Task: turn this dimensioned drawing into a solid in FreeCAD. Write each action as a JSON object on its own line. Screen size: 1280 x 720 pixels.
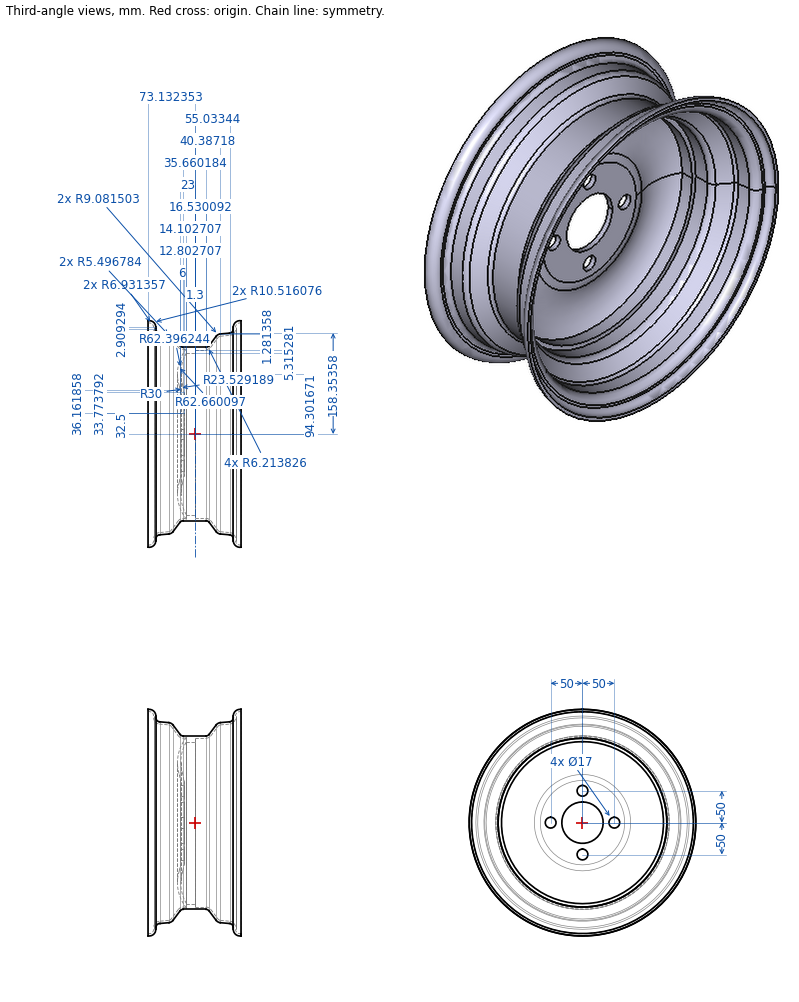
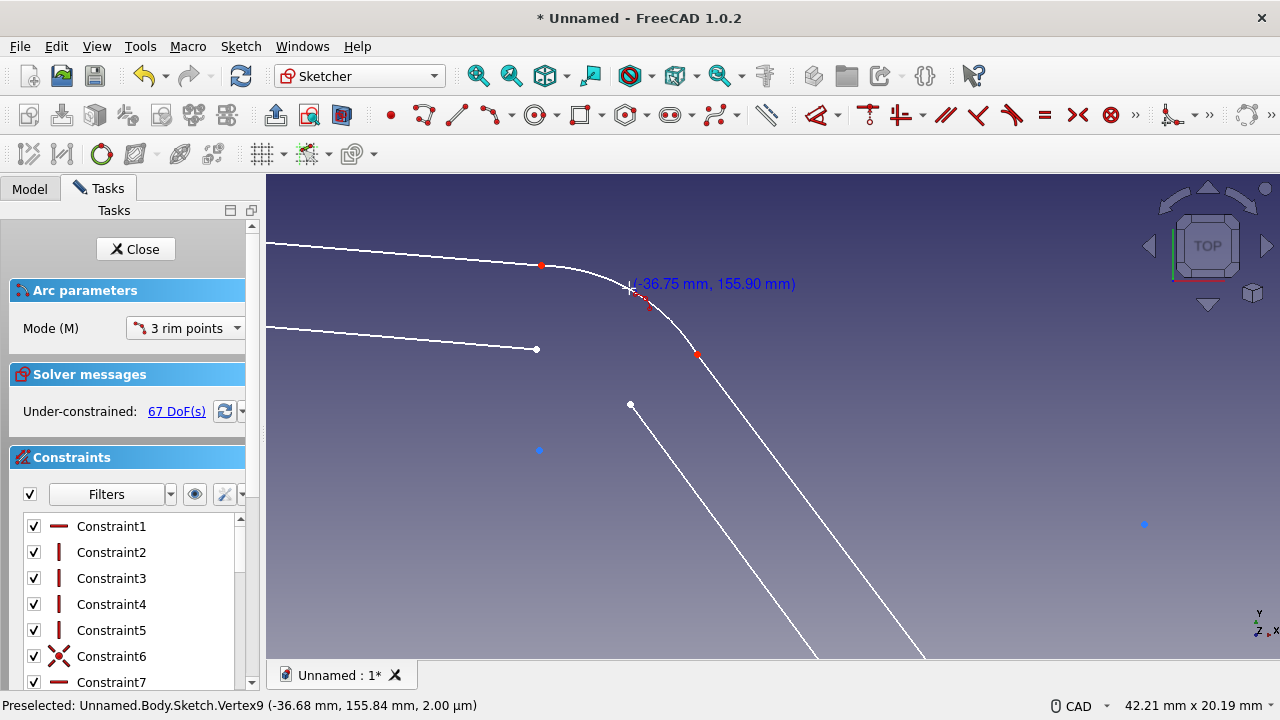
{"action": "scroll", "coordinate": [640, 298], "scroll_direction": "down", "scroll_amount": 13}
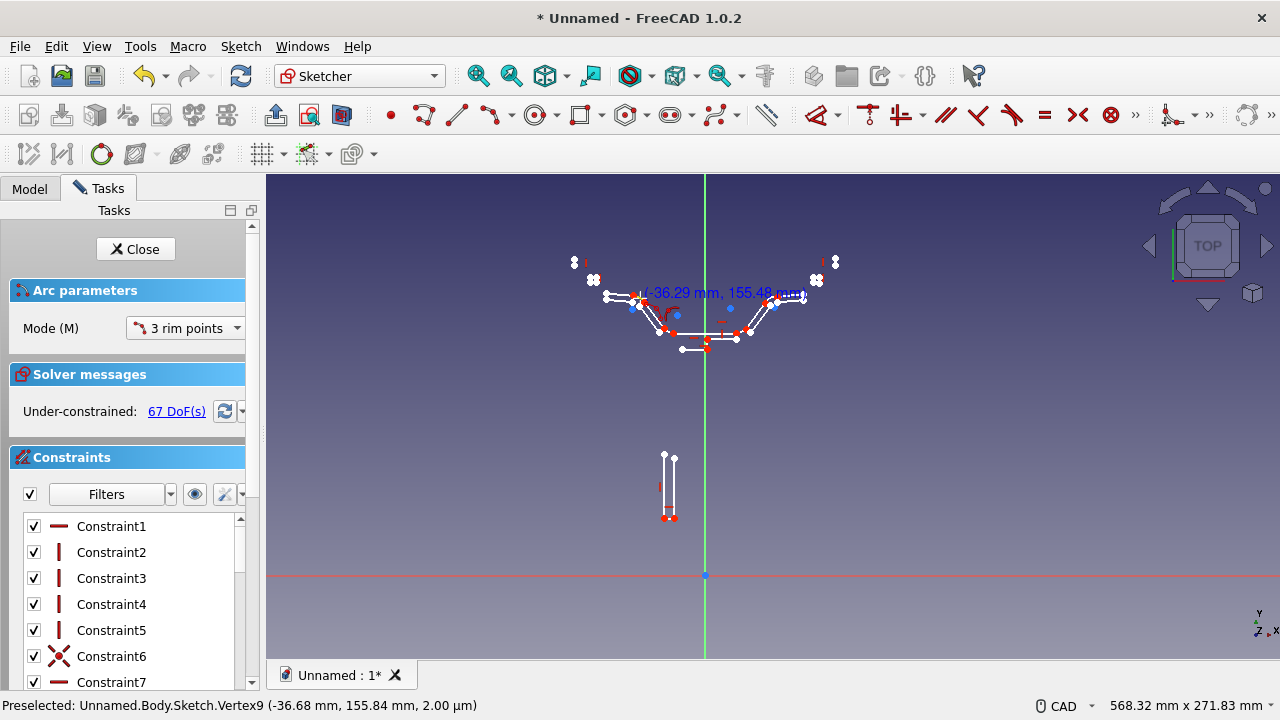
{"action": "scroll", "coordinate": [607, 293], "scroll_direction": "up", "scroll_amount": 5}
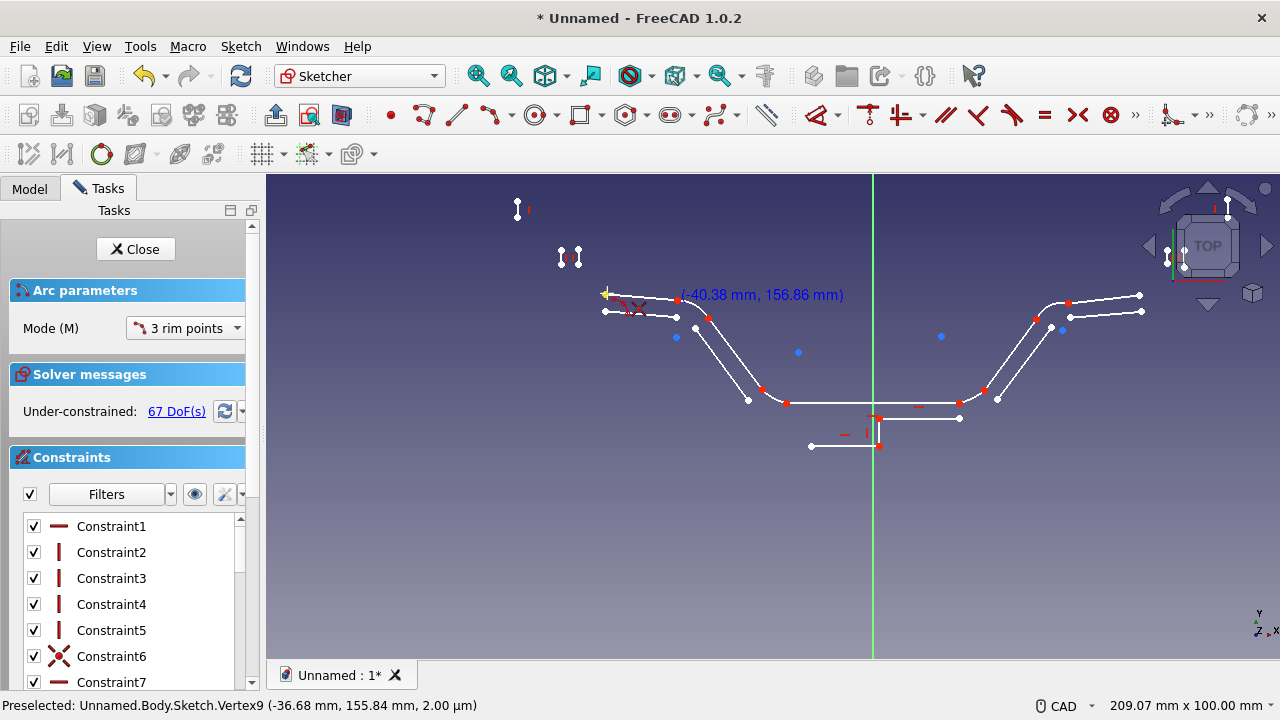
{"action": "left_click", "coordinate": [606, 294]}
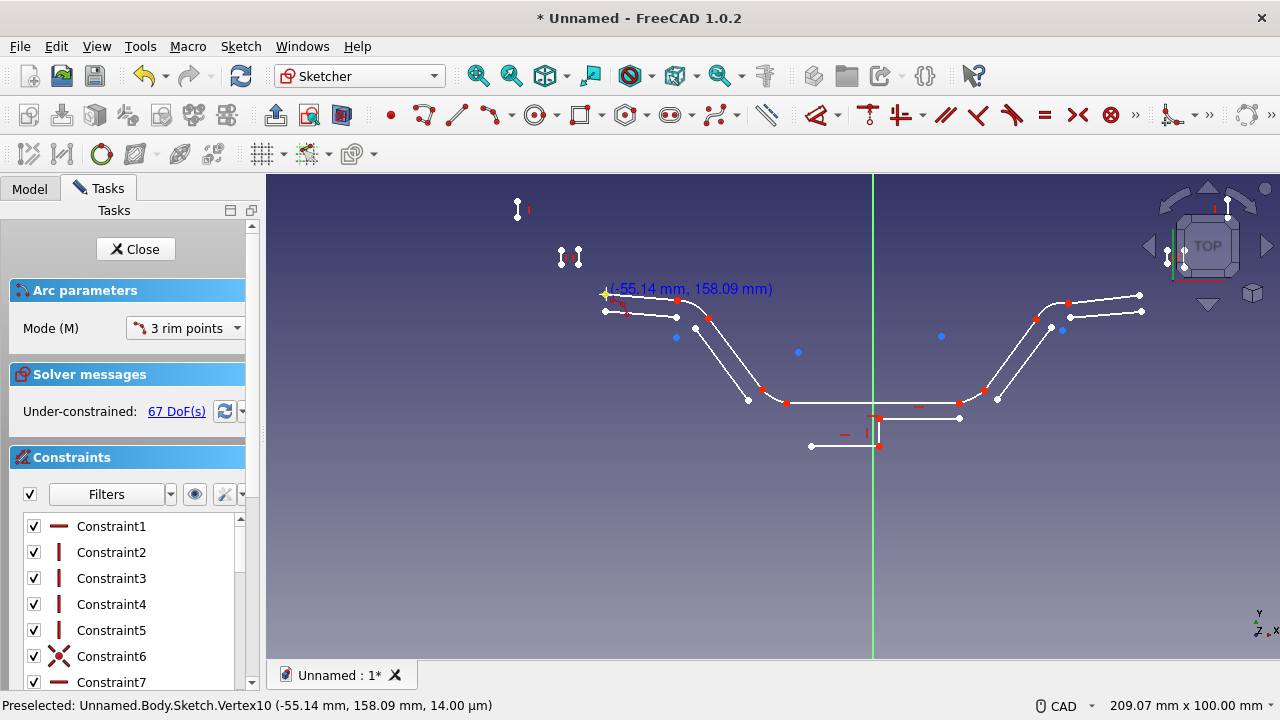
{"action": "scroll", "coordinate": [579, 263], "scroll_direction": "up", "scroll_amount": 5}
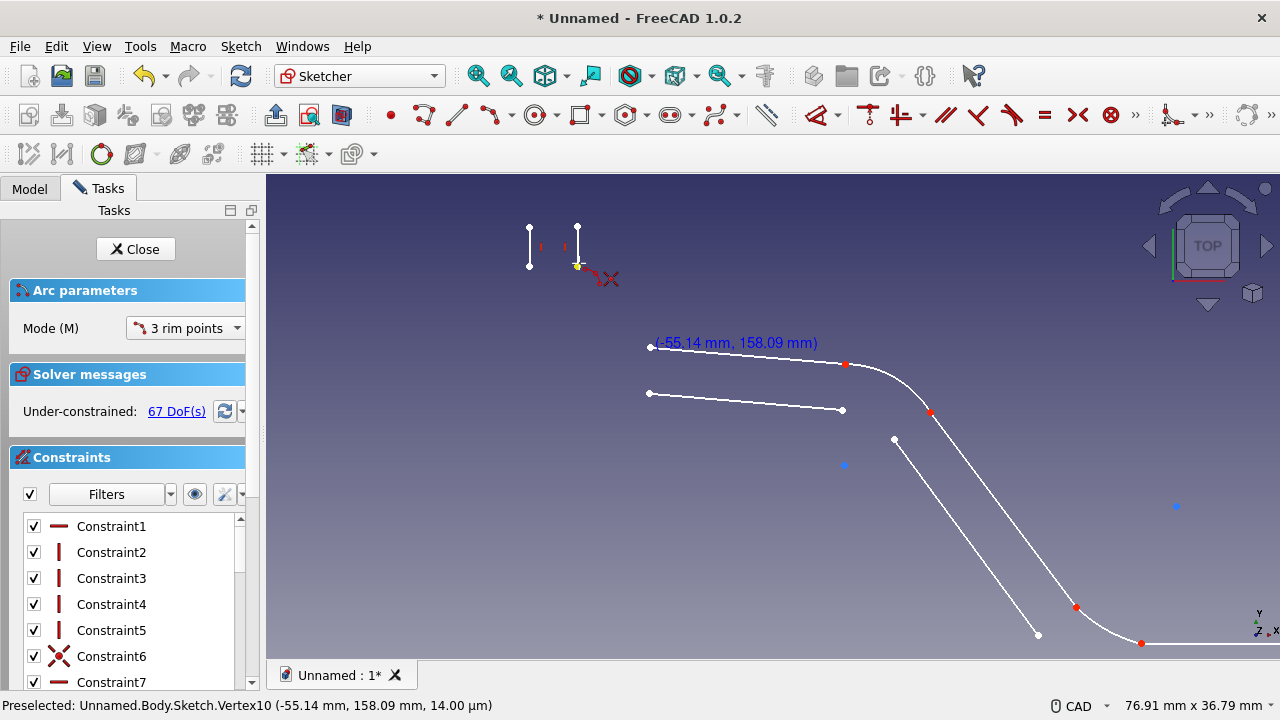
{"action": "left_click", "coordinate": [578, 267]}
{"action": "left_click", "coordinate": [599, 318]}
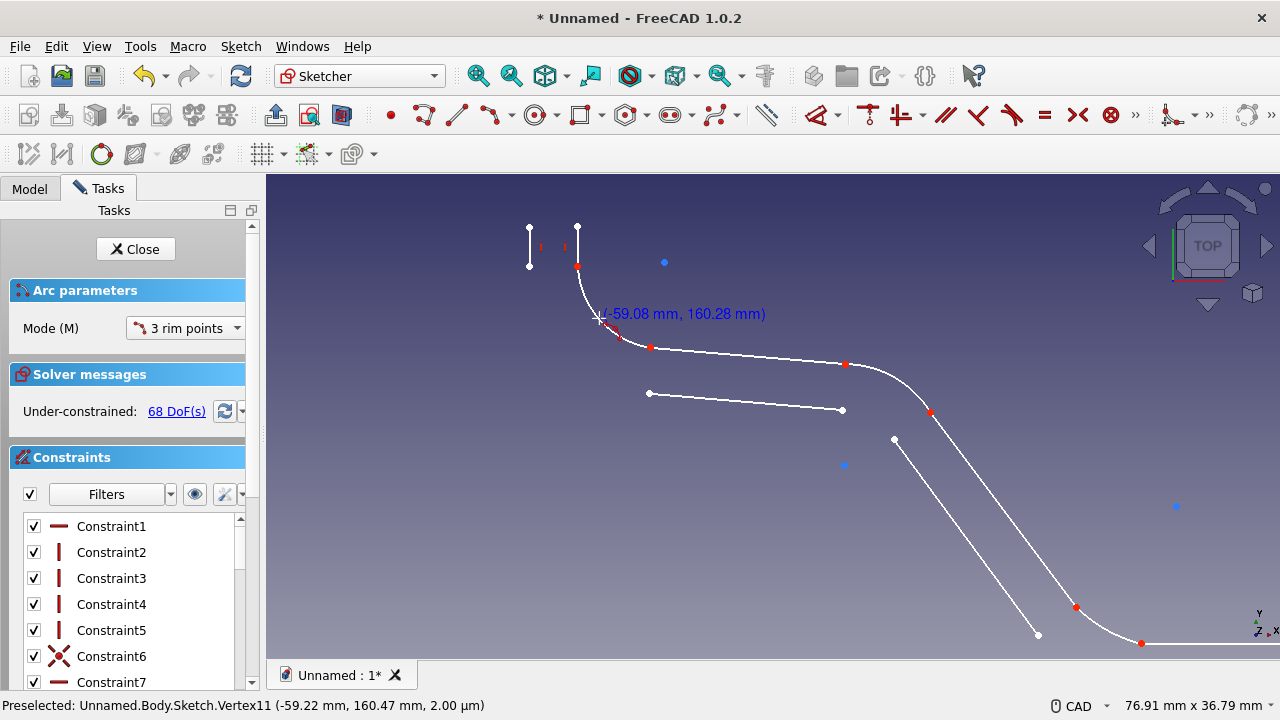
{"action": "left_click", "coordinate": [578, 226]}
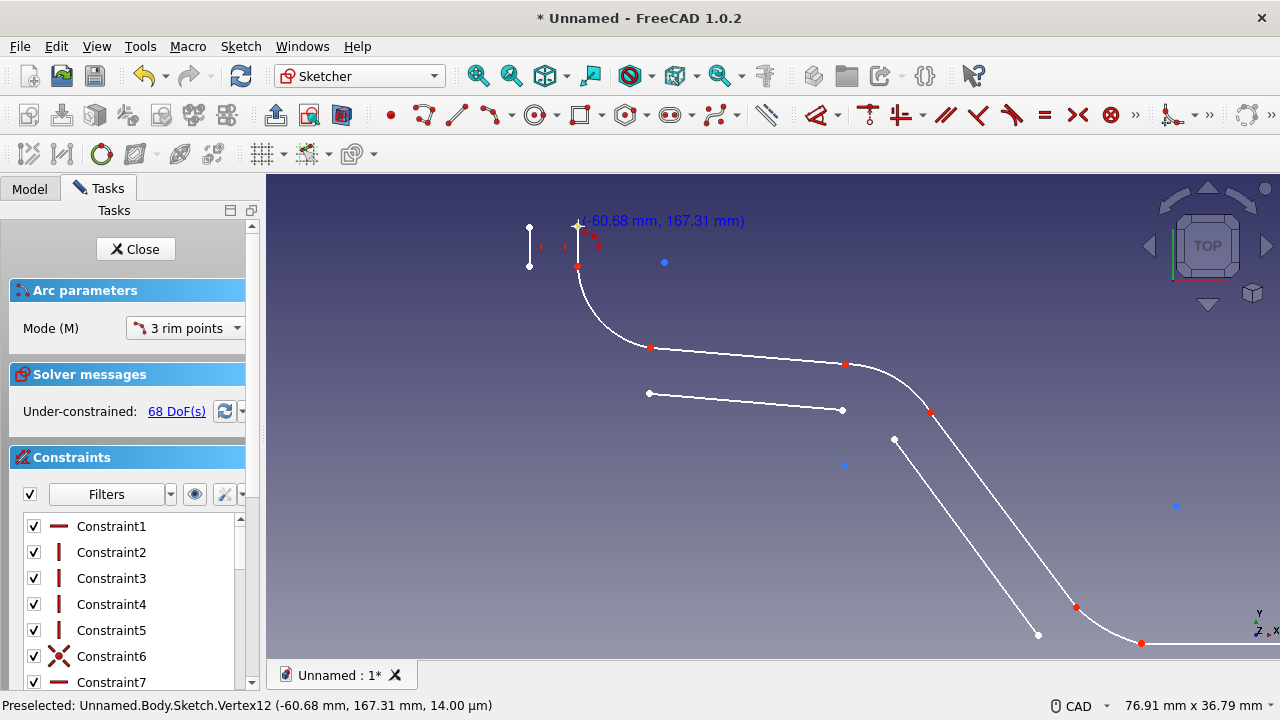
{"action": "scroll", "coordinate": [599, 284], "scroll_direction": "down", "scroll_amount": 10}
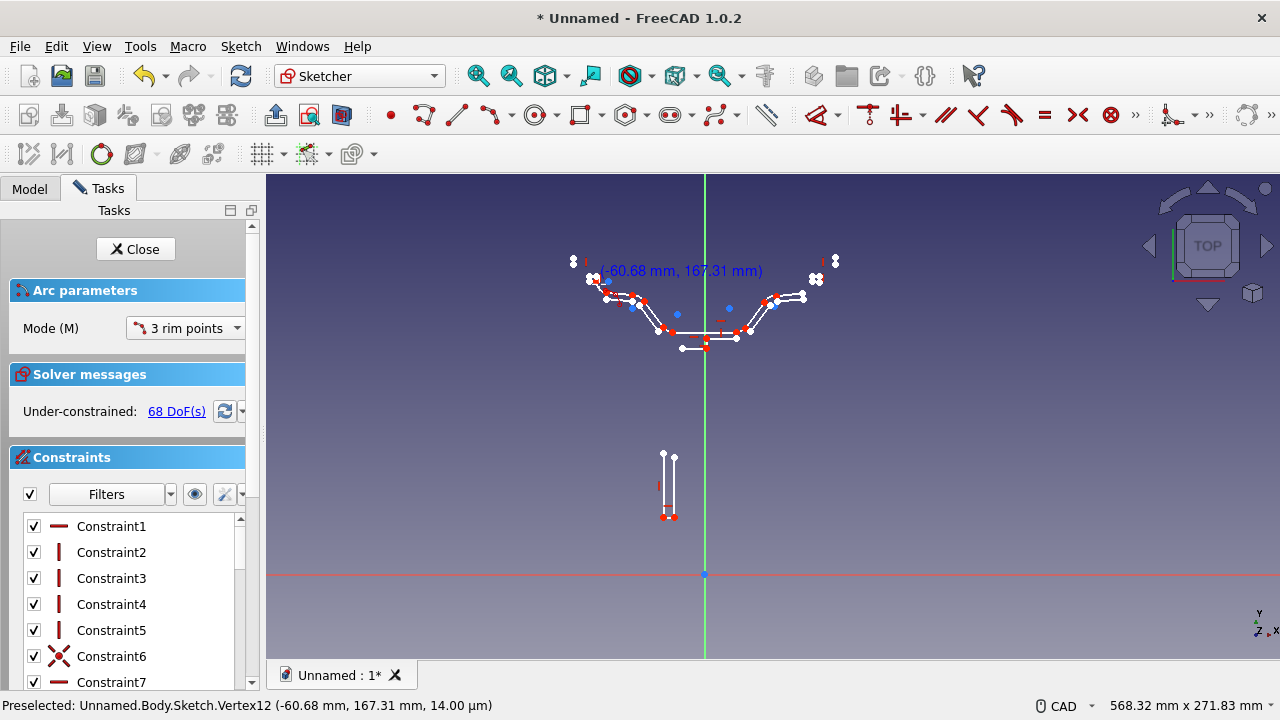
{"action": "scroll", "coordinate": [574, 258], "scroll_direction": "up", "scroll_amount": 8}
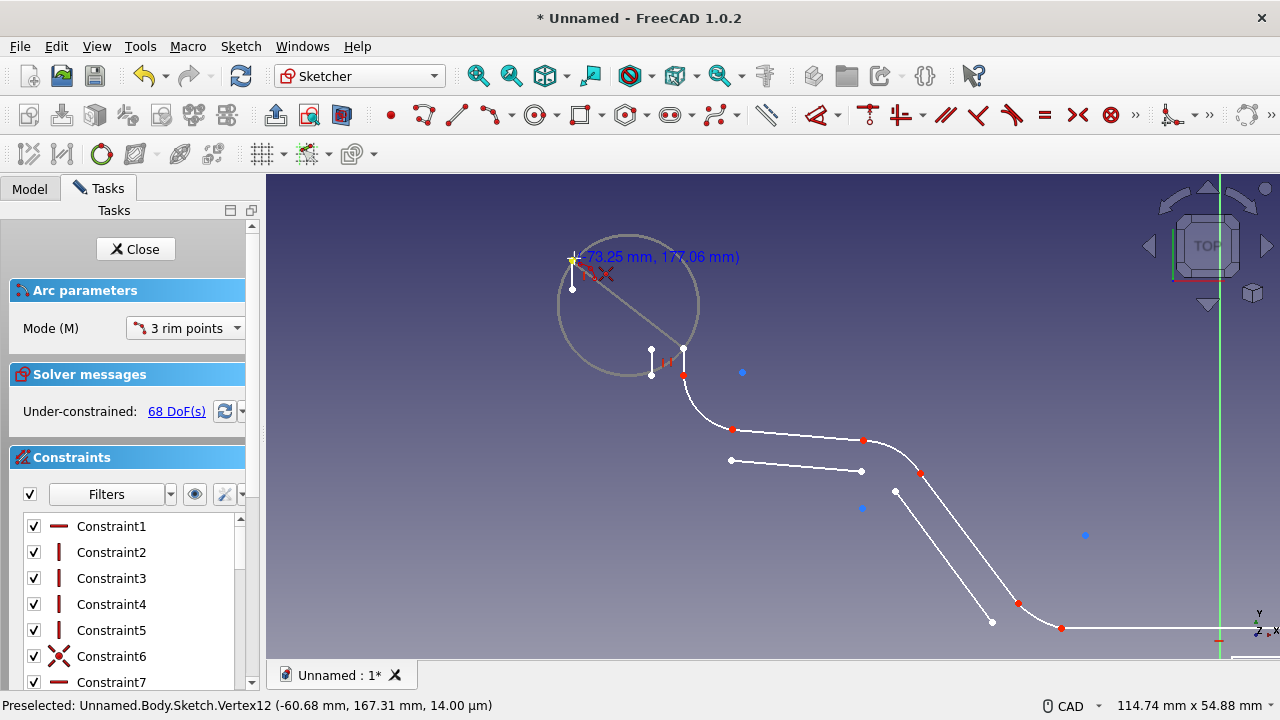
{"action": "left_click", "coordinate": [572, 261]}
{"action": "left_click", "coordinate": [650, 276]}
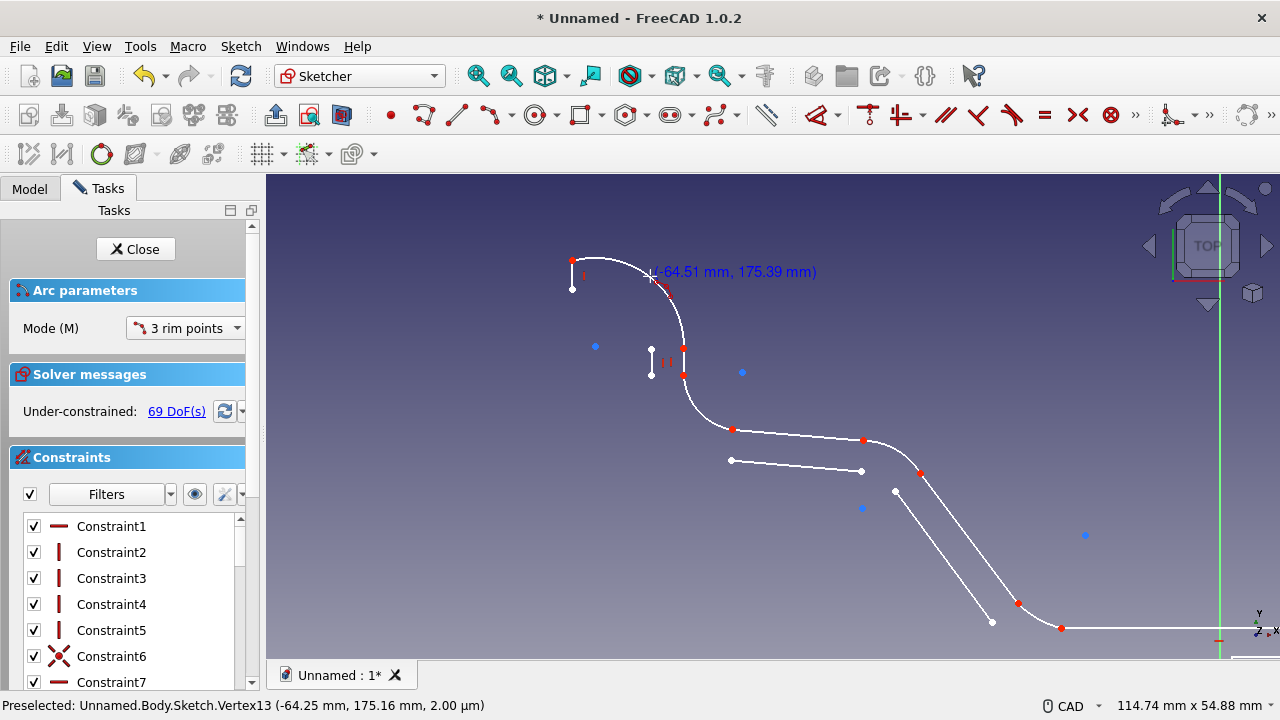
{"action": "left_click", "coordinate": [572, 289]}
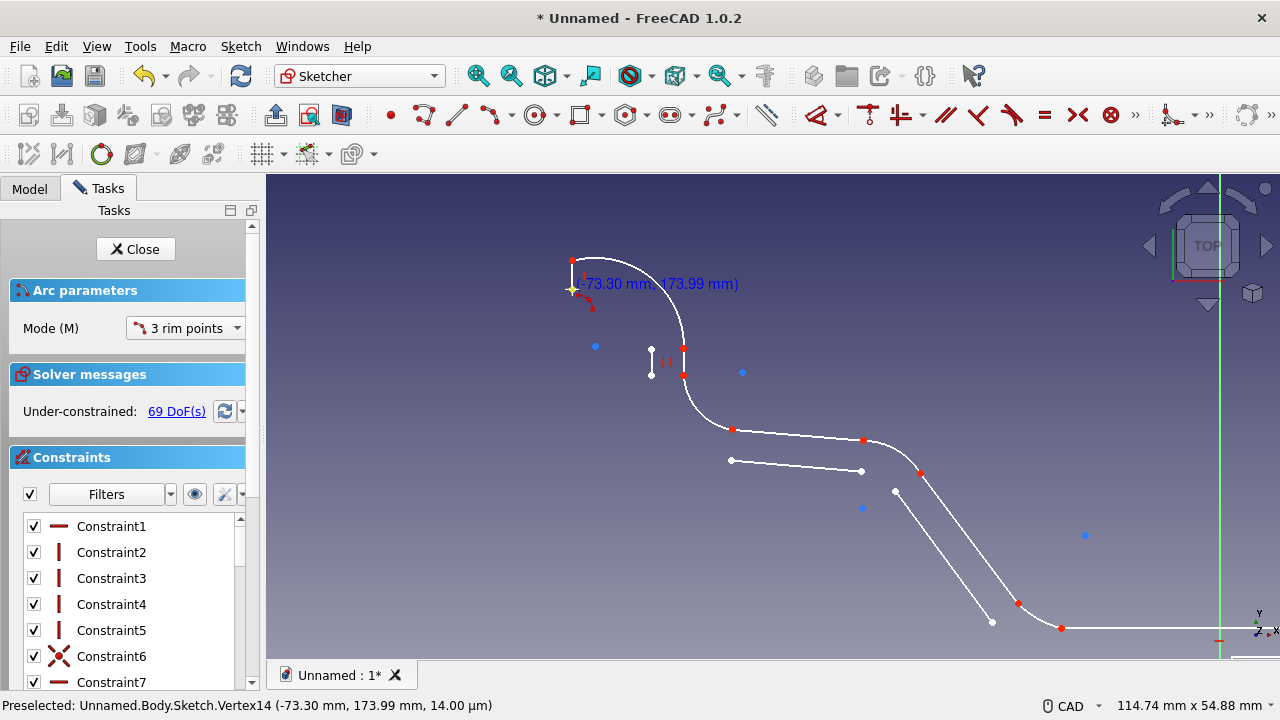
{"action": "scroll", "coordinate": [652, 347], "scroll_direction": "up", "scroll_amount": 2}